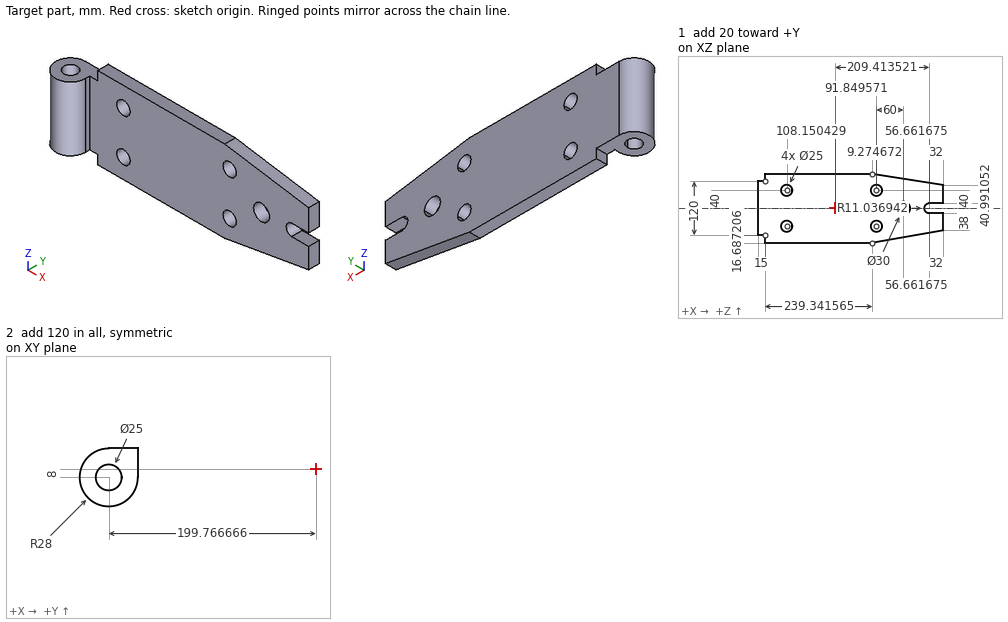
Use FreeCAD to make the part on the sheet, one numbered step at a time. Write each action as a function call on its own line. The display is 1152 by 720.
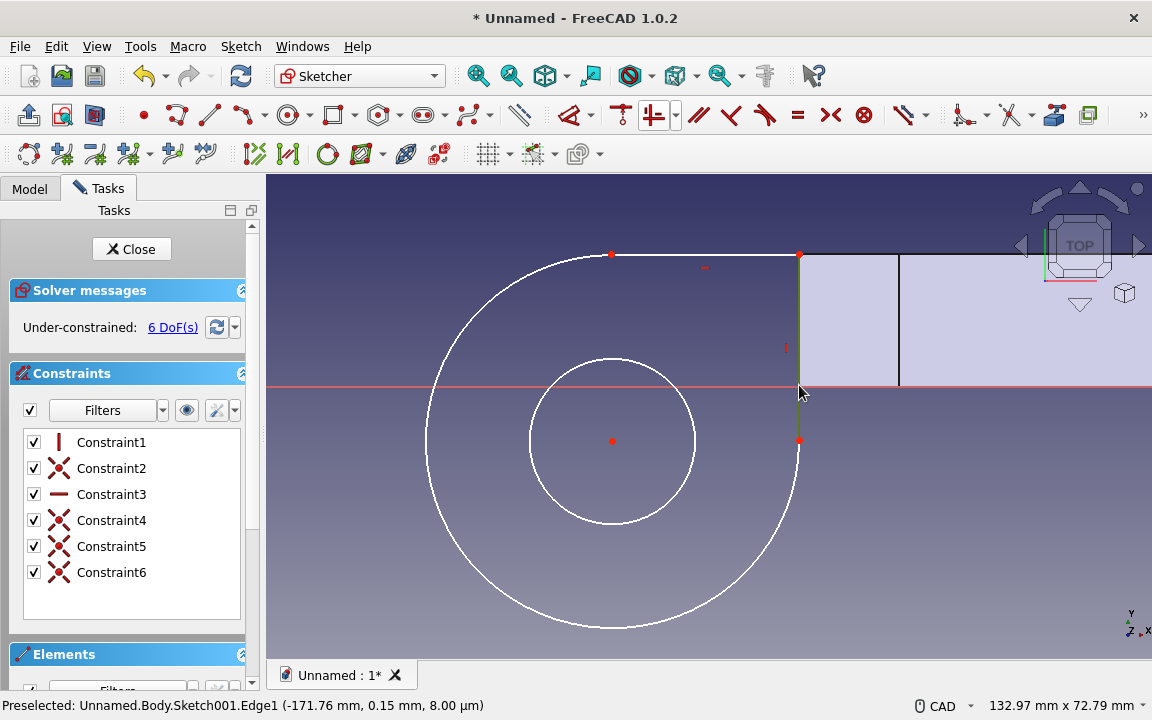
click(428, 413)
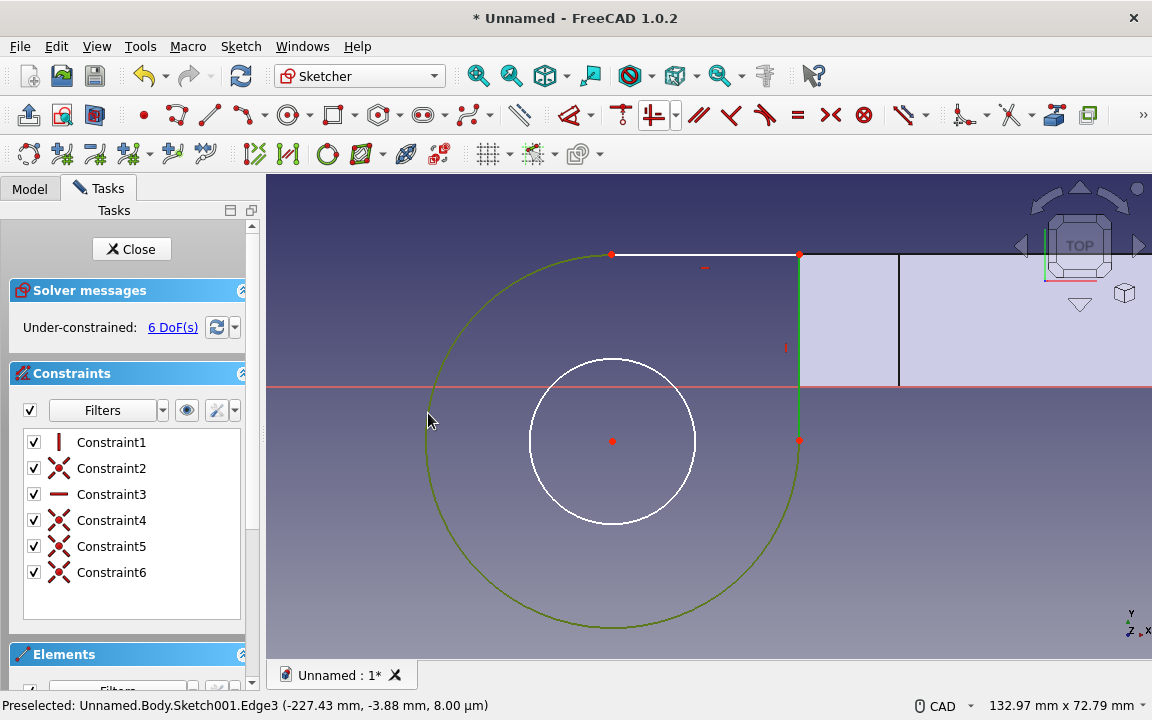
key(t)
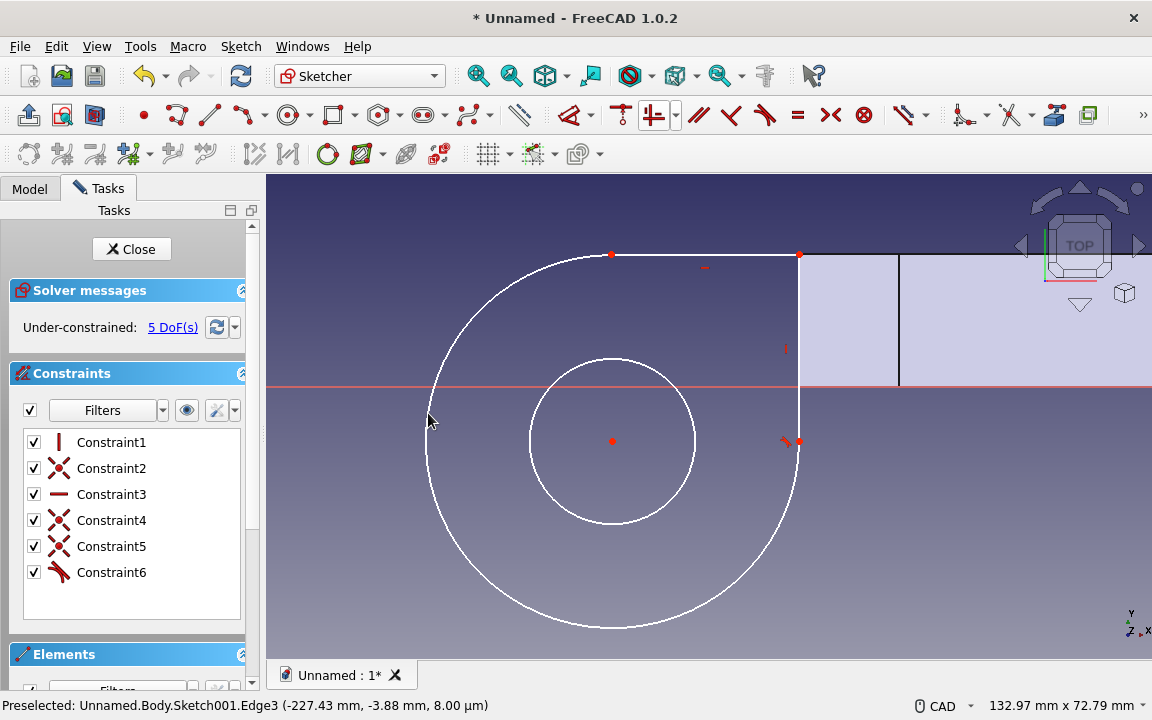
click(743, 255)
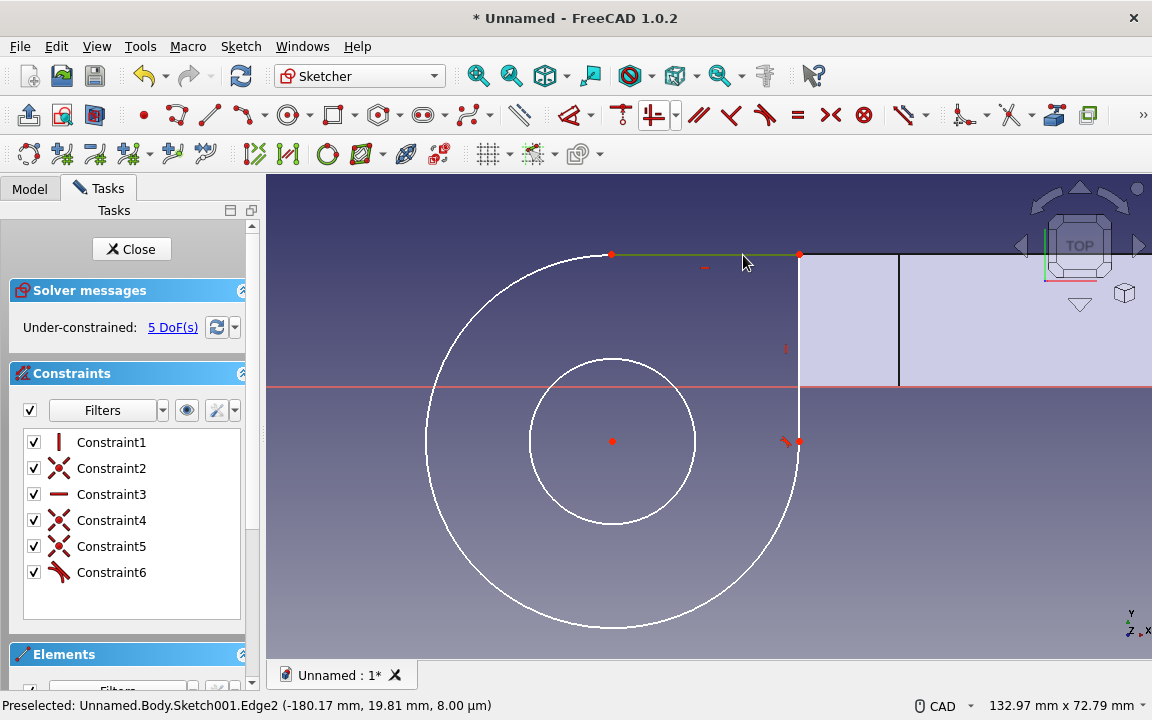
click(428, 413)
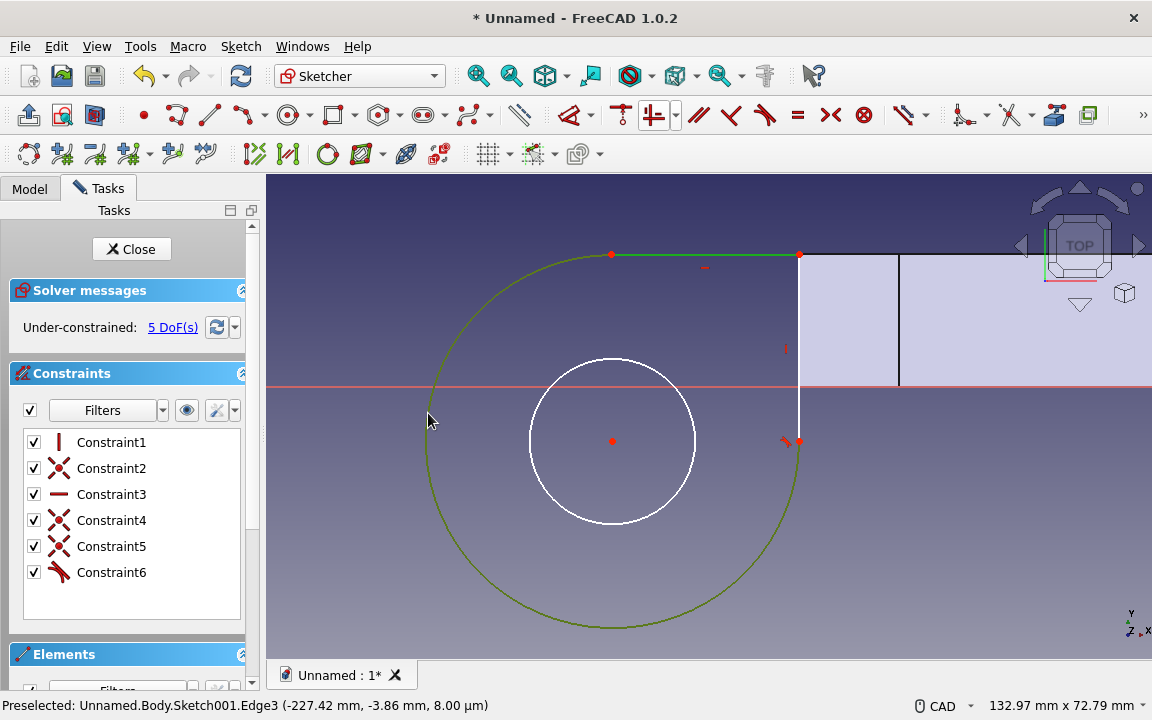
click(765, 116)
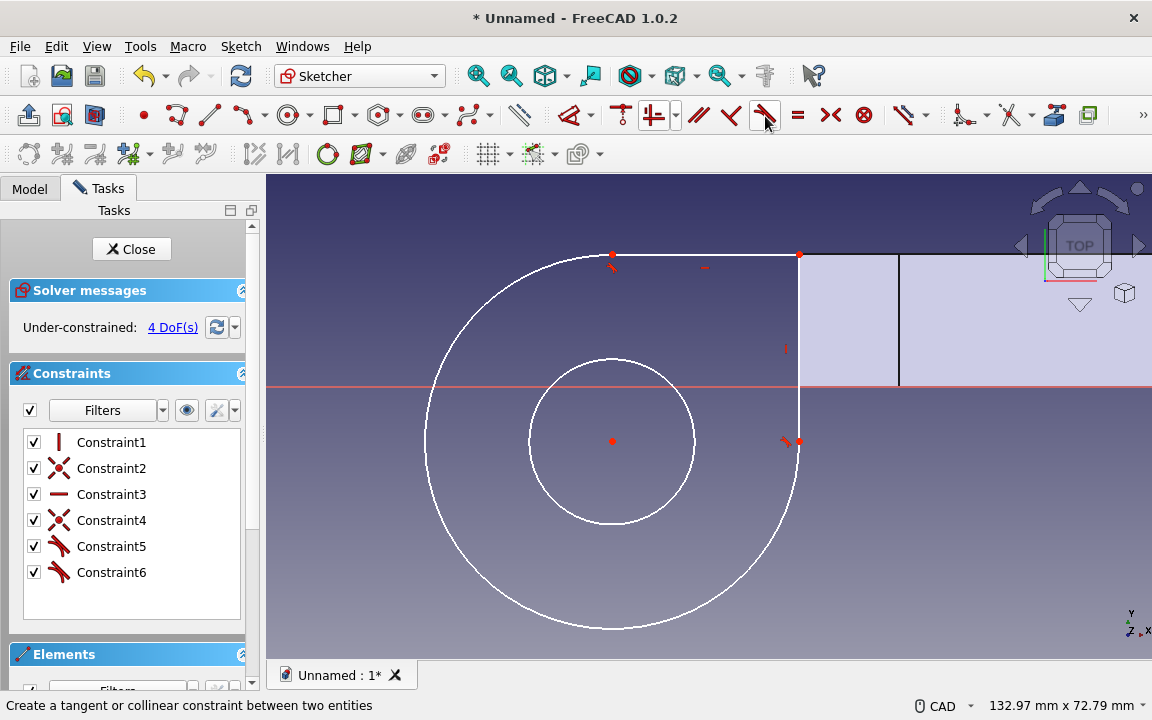
click(568, 116)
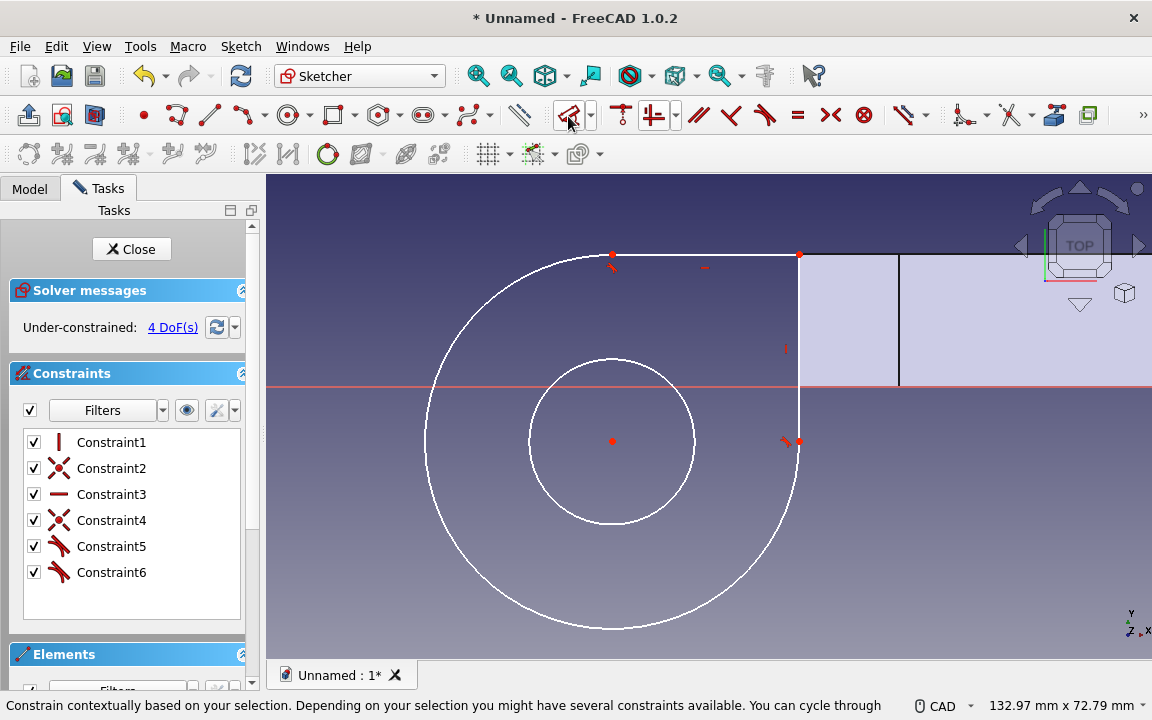
click(427, 413)
click(395, 408)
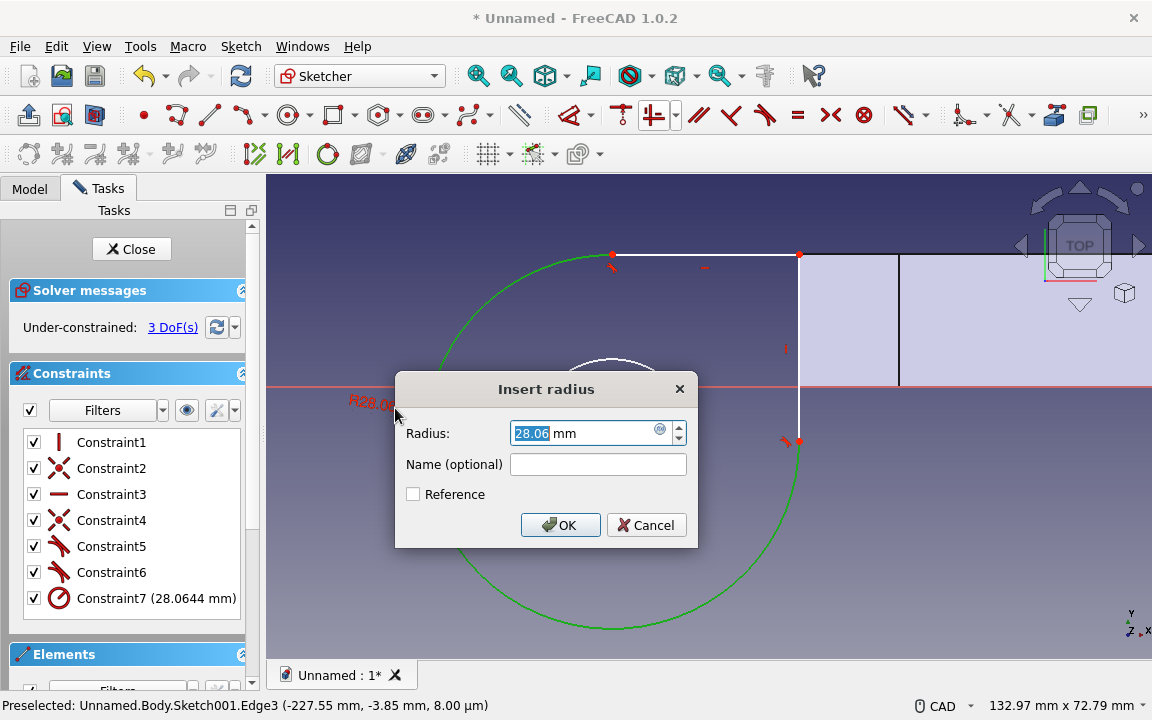
text(28)
key(Return)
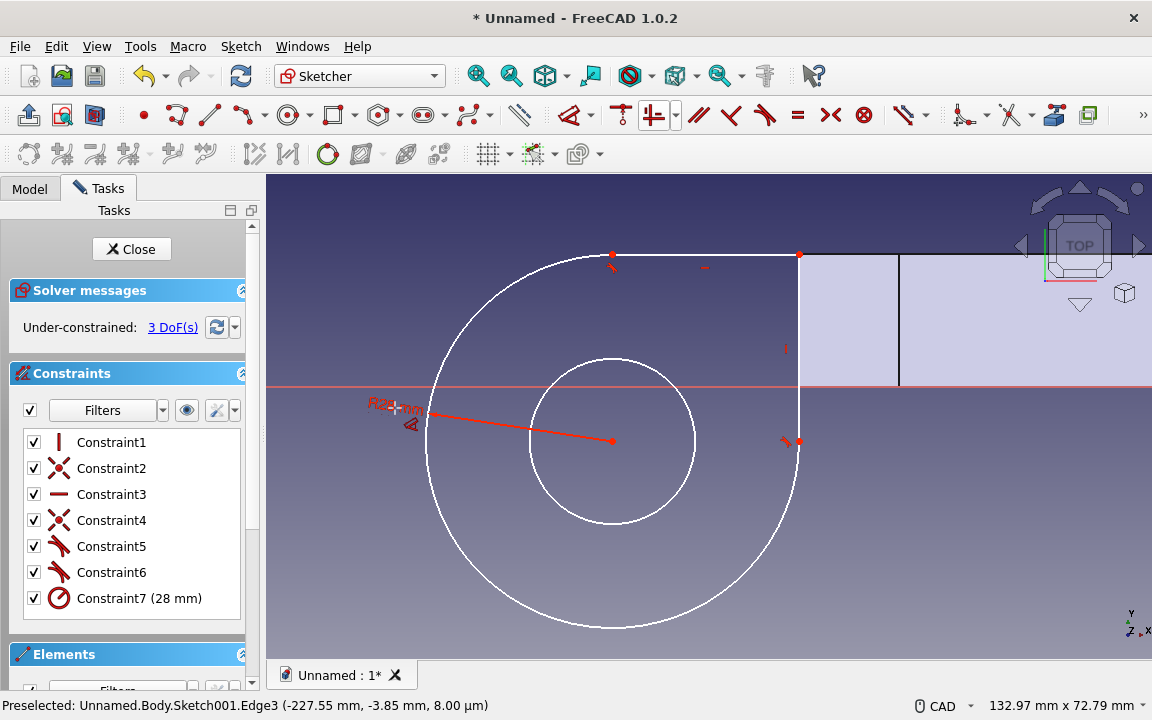
click(554, 383)
click(531, 360)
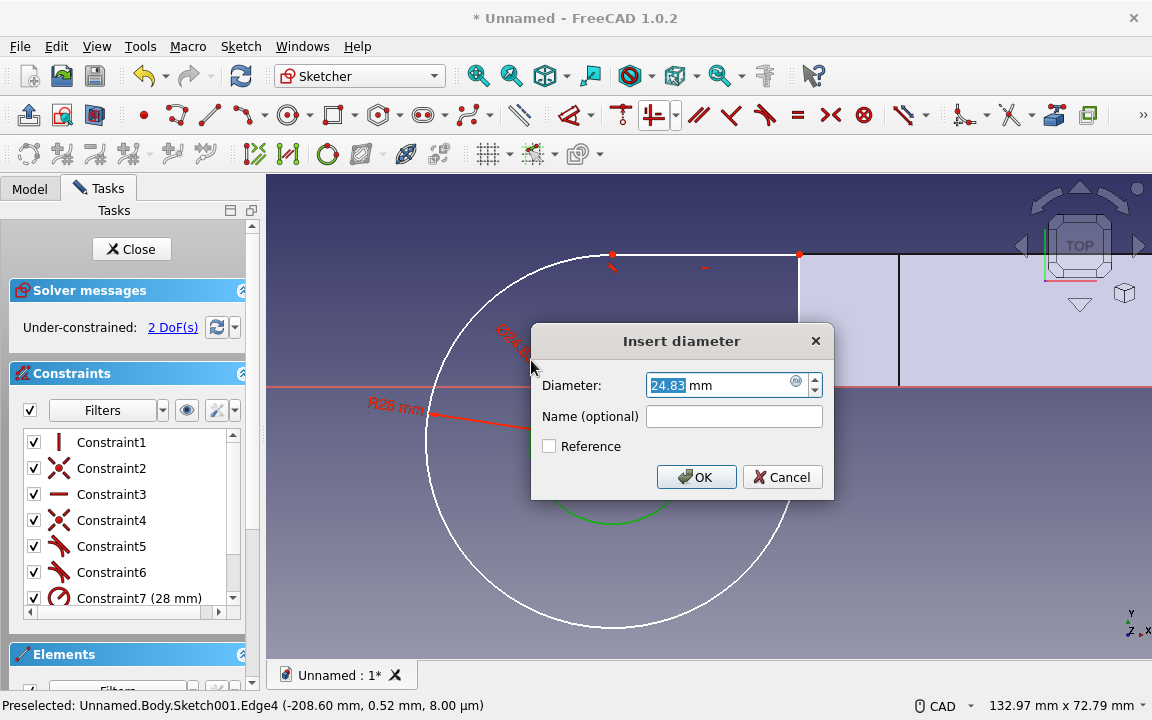
text(25)
key(Return)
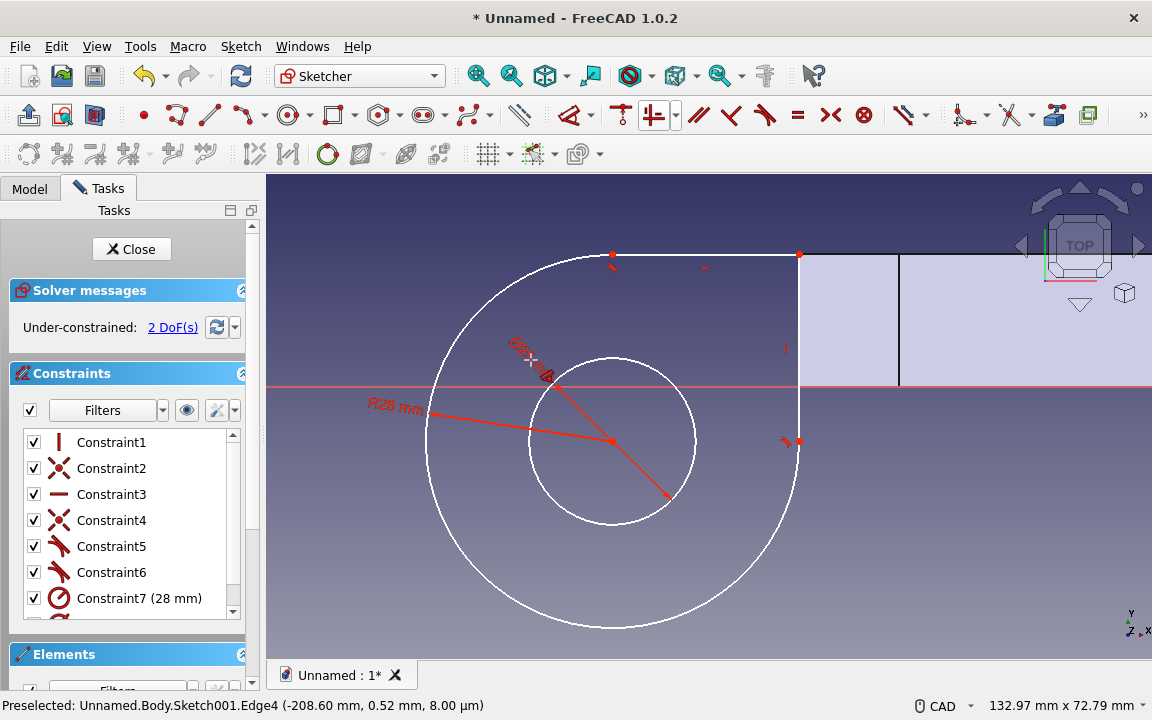
click(612, 441)
click(578, 414)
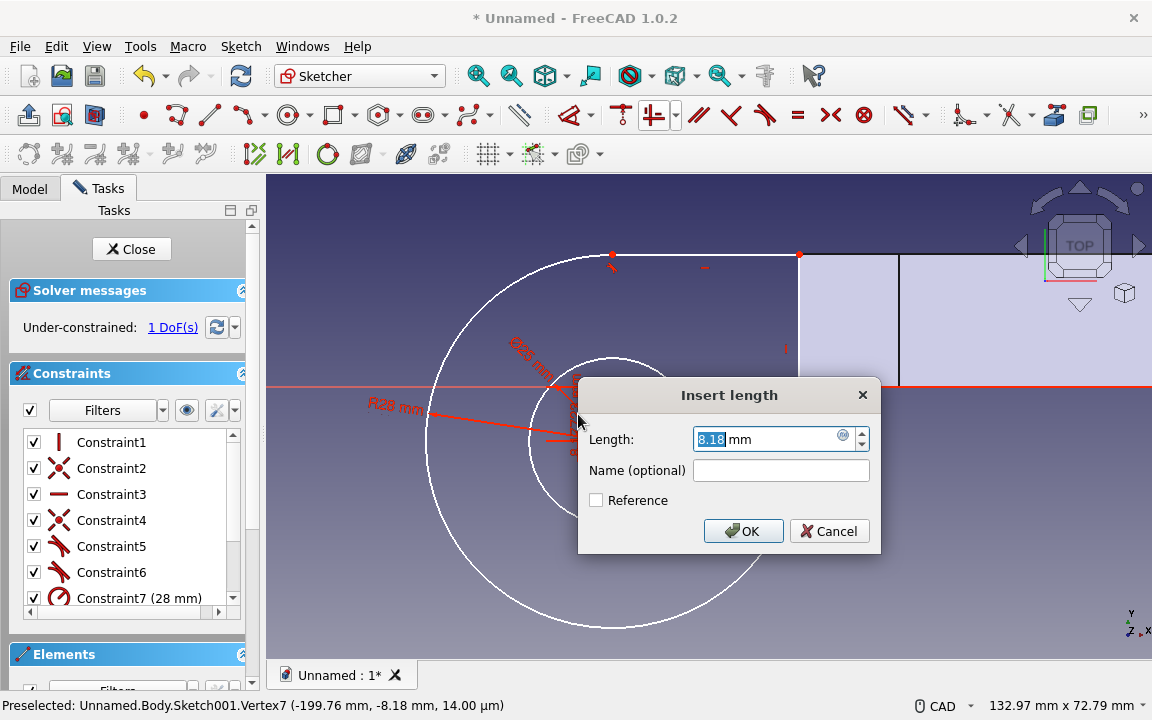
text(8)
key(Return)